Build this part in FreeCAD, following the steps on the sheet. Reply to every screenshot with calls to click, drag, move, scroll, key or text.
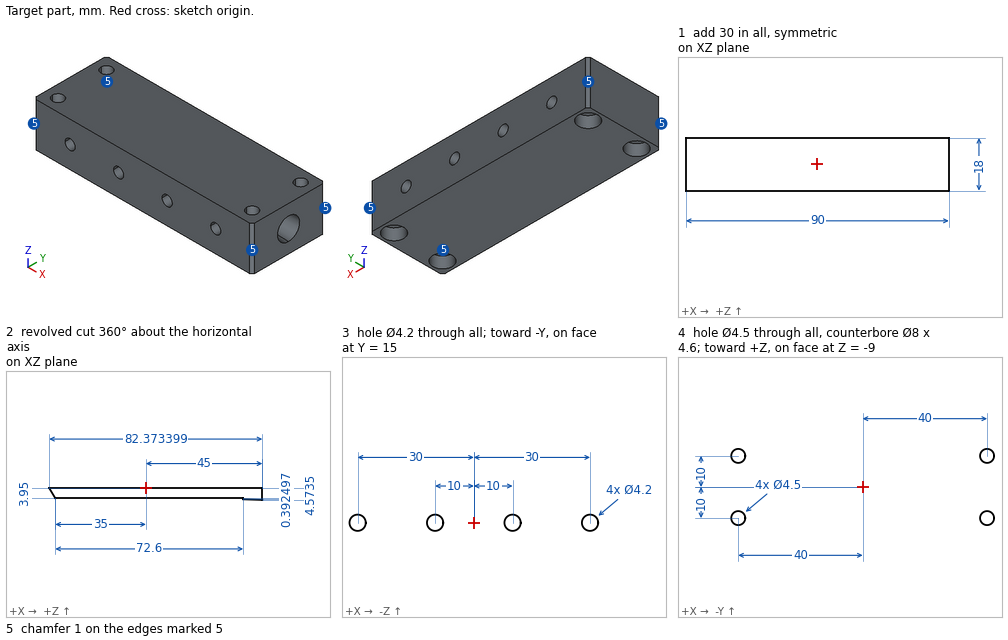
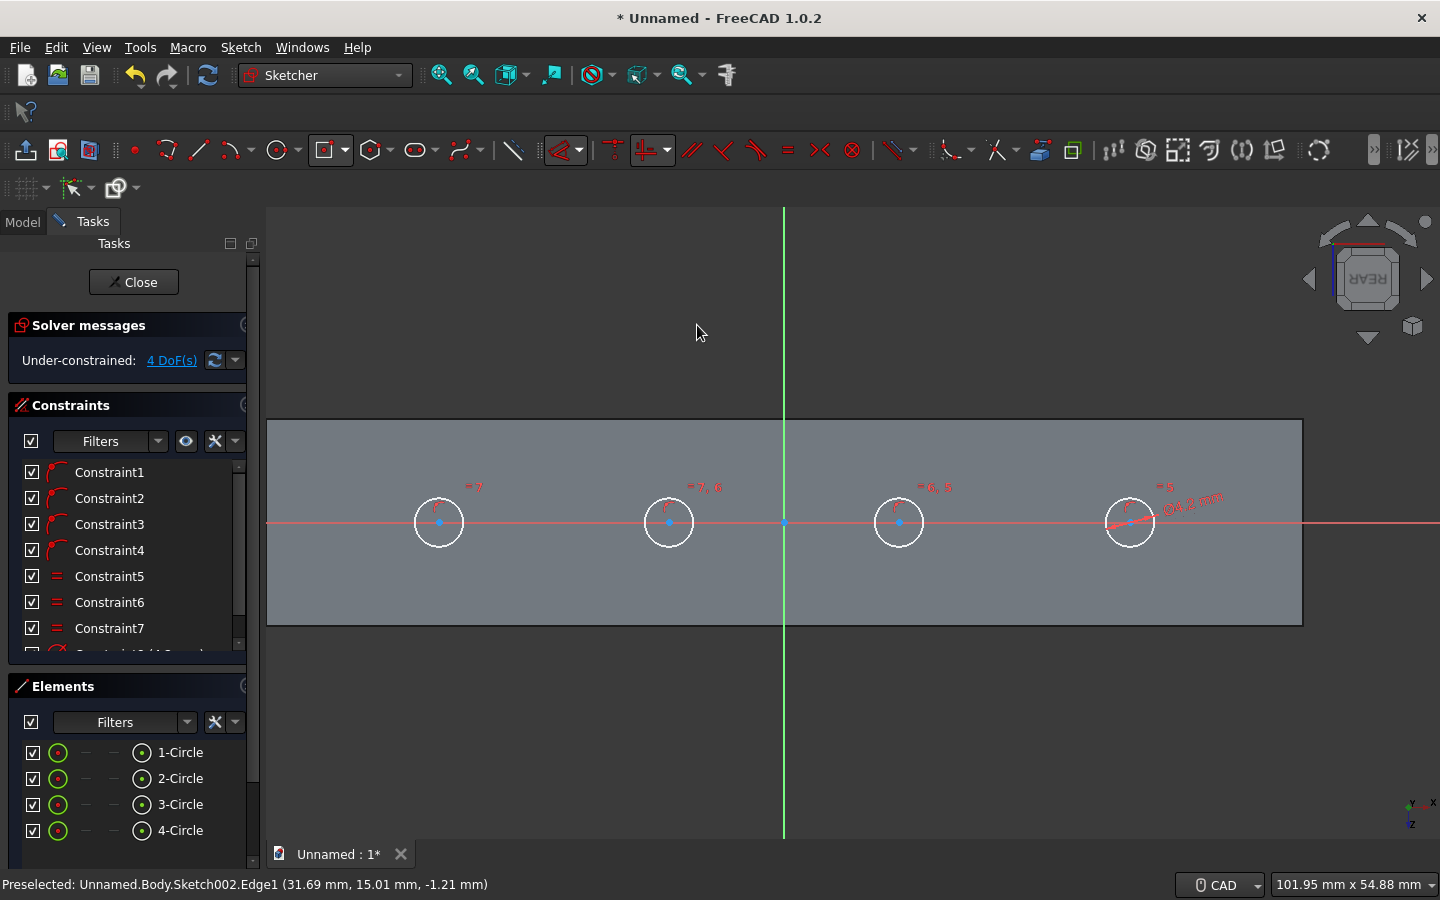
click(1130, 523)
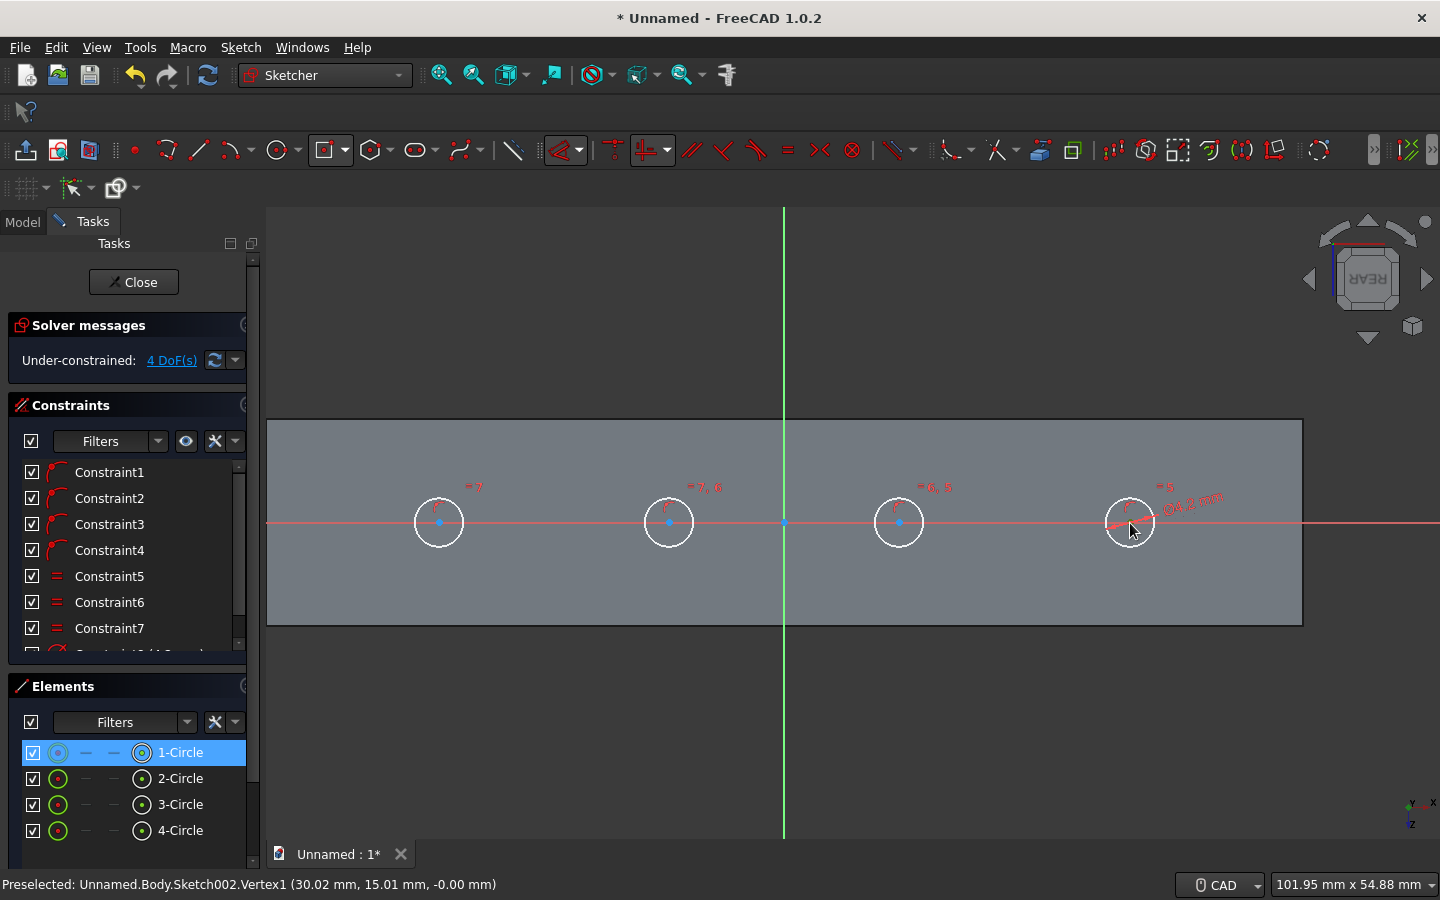
key(l)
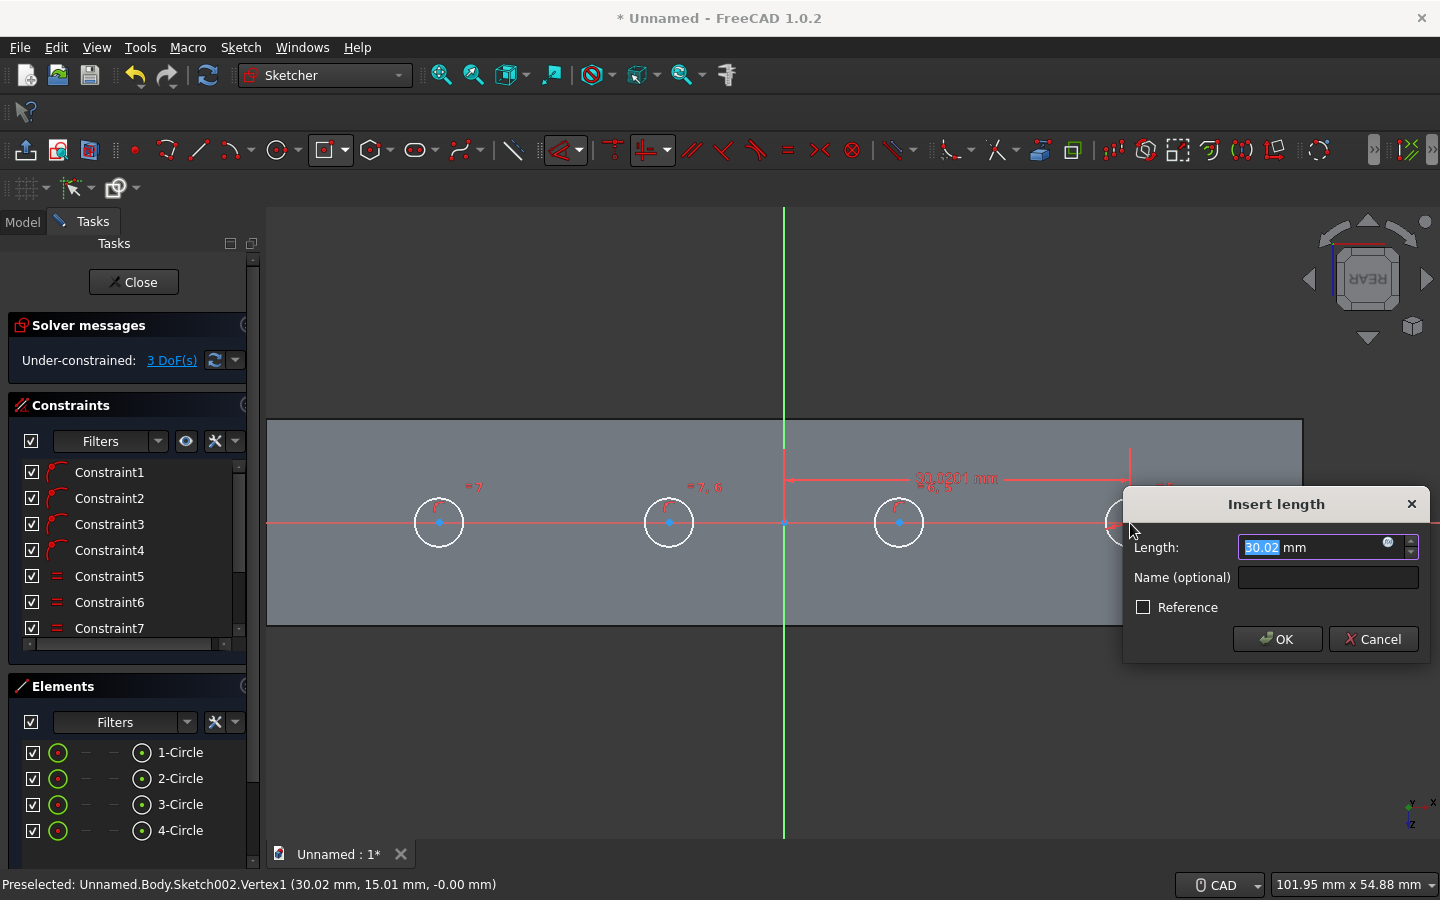
text(30)
key(Return)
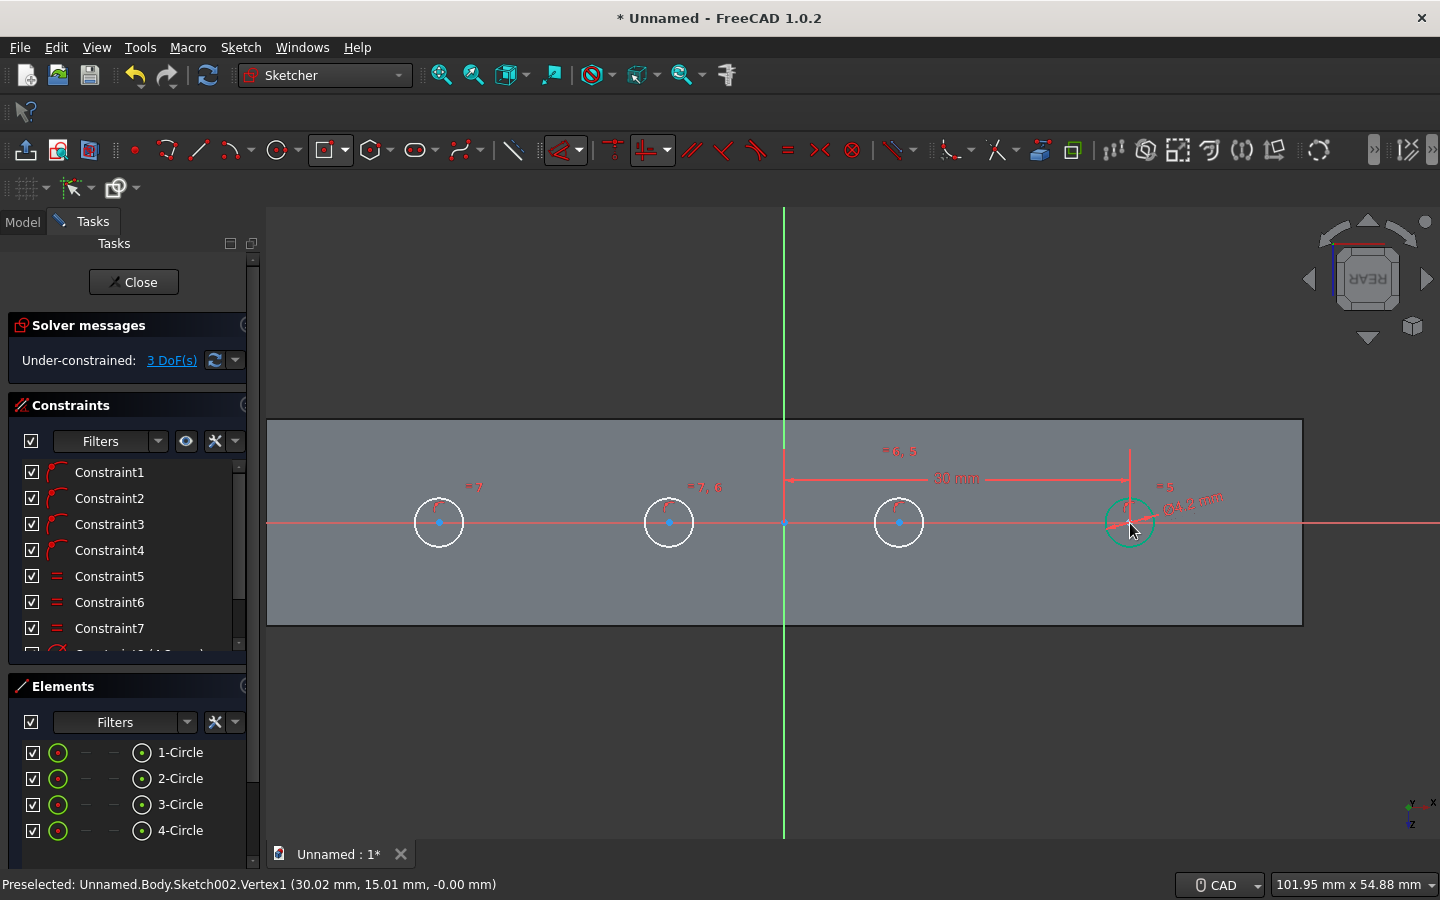
click(899, 523)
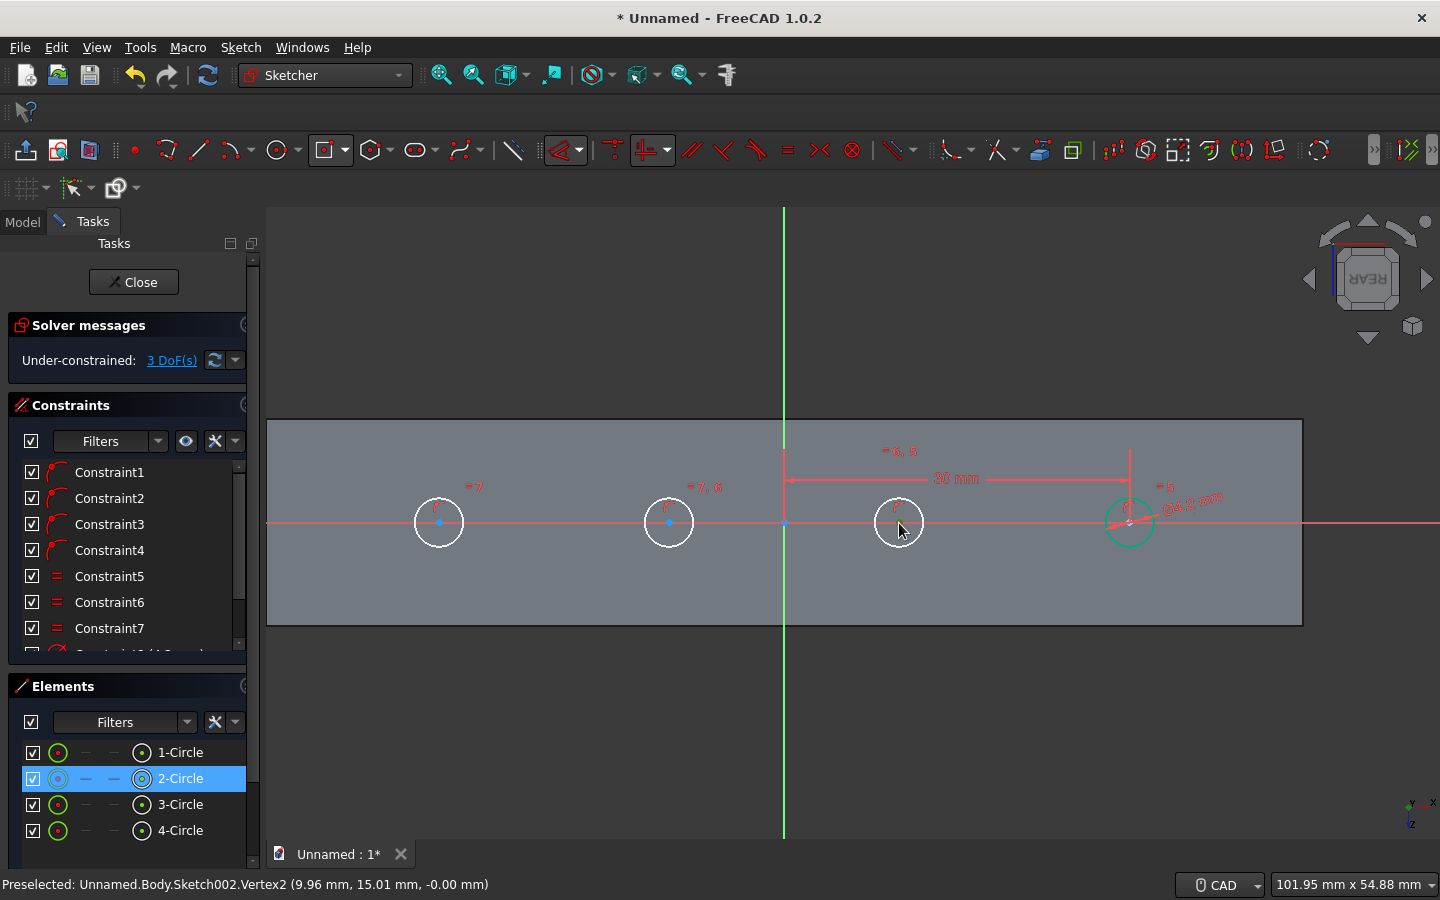
click(582, 150)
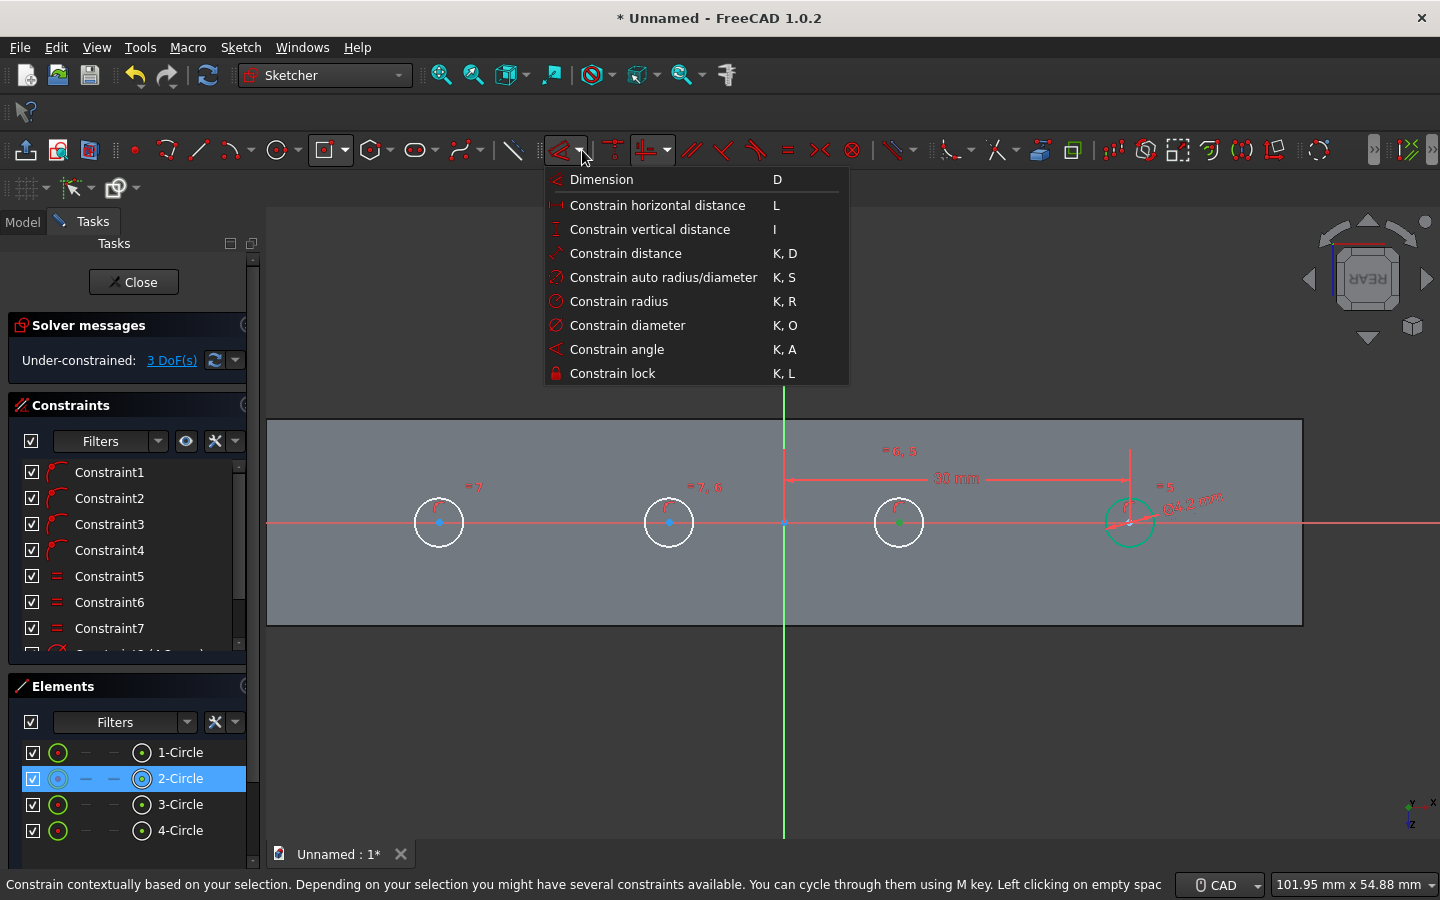
click(697, 205)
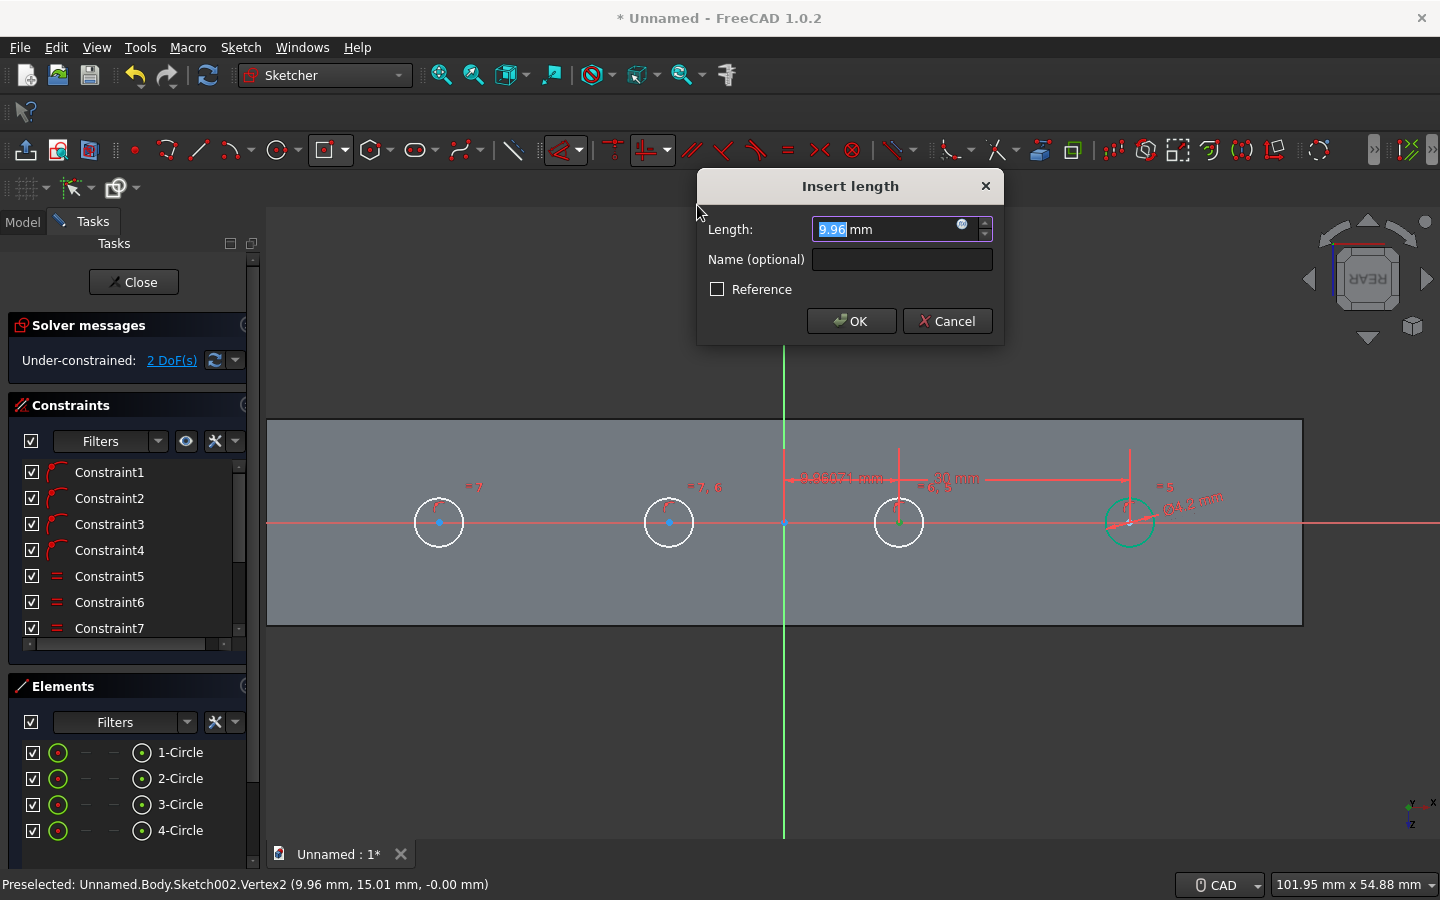
text(10)
key(Return)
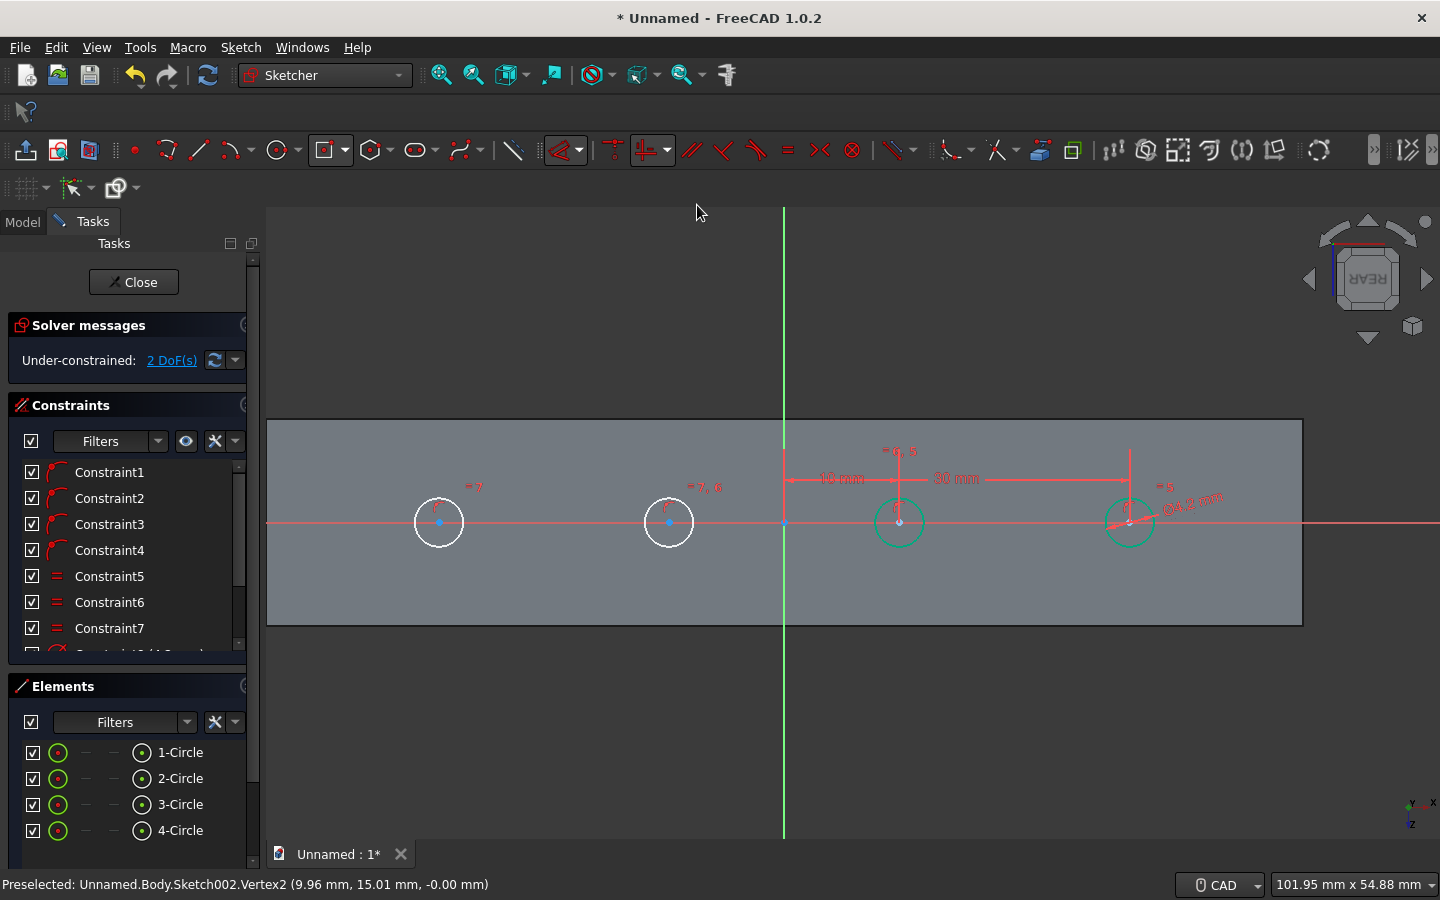
click(669, 523)